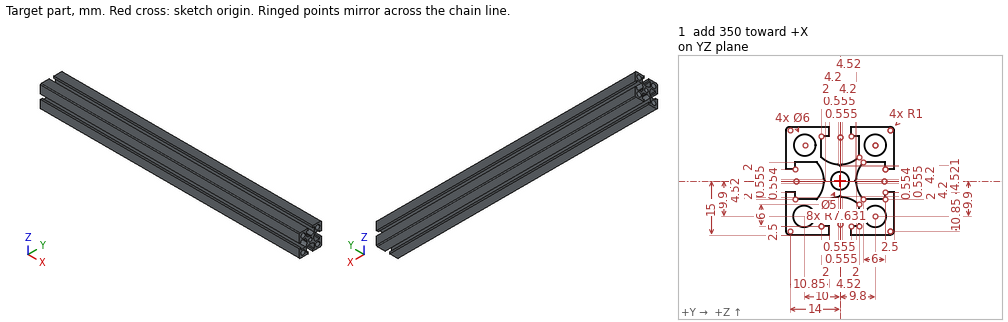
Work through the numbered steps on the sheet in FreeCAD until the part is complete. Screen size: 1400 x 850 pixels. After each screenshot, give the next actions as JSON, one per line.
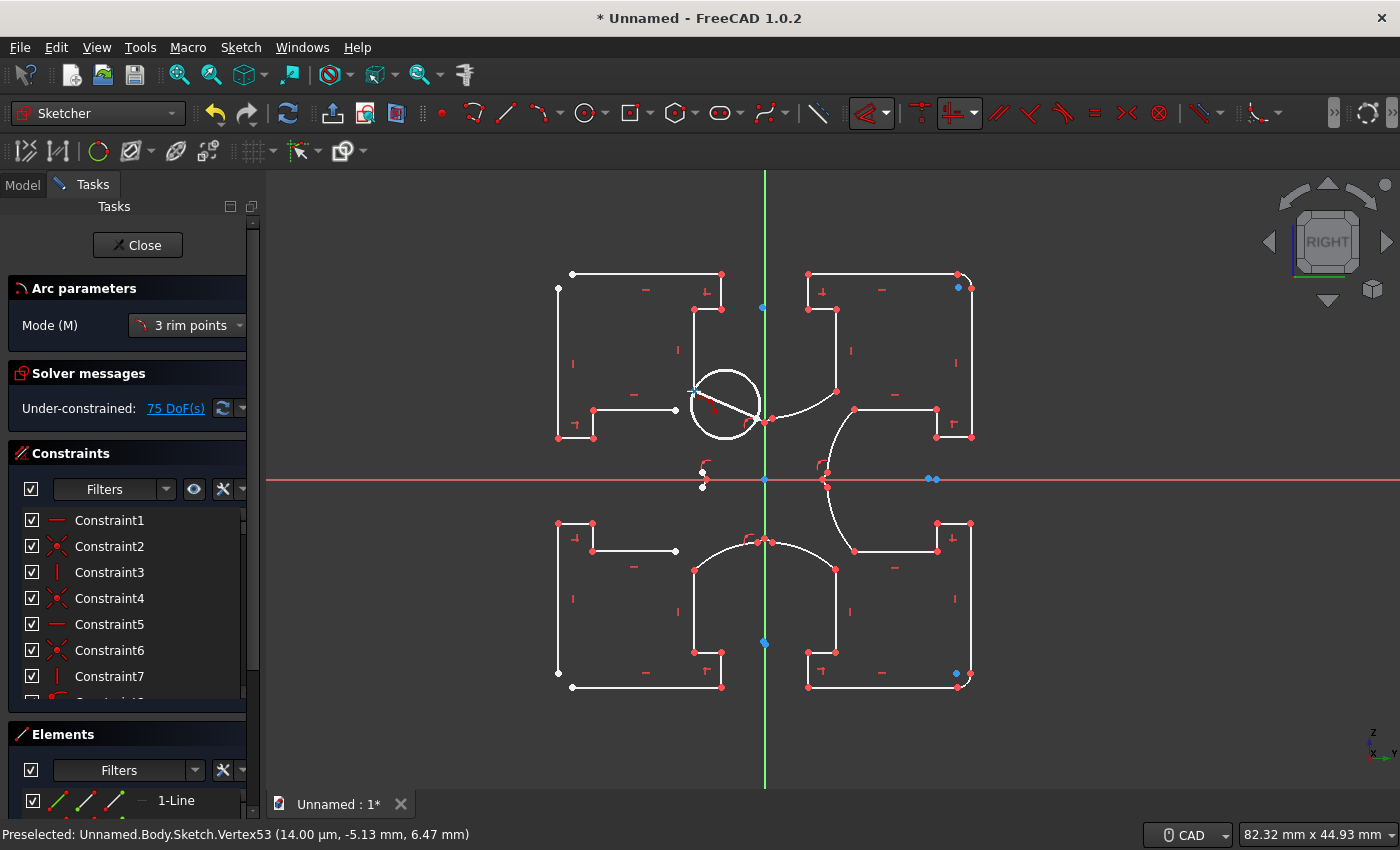
{"action": "scroll", "coordinate": [723, 409], "scroll_direction": "up", "scroll_amount": 6}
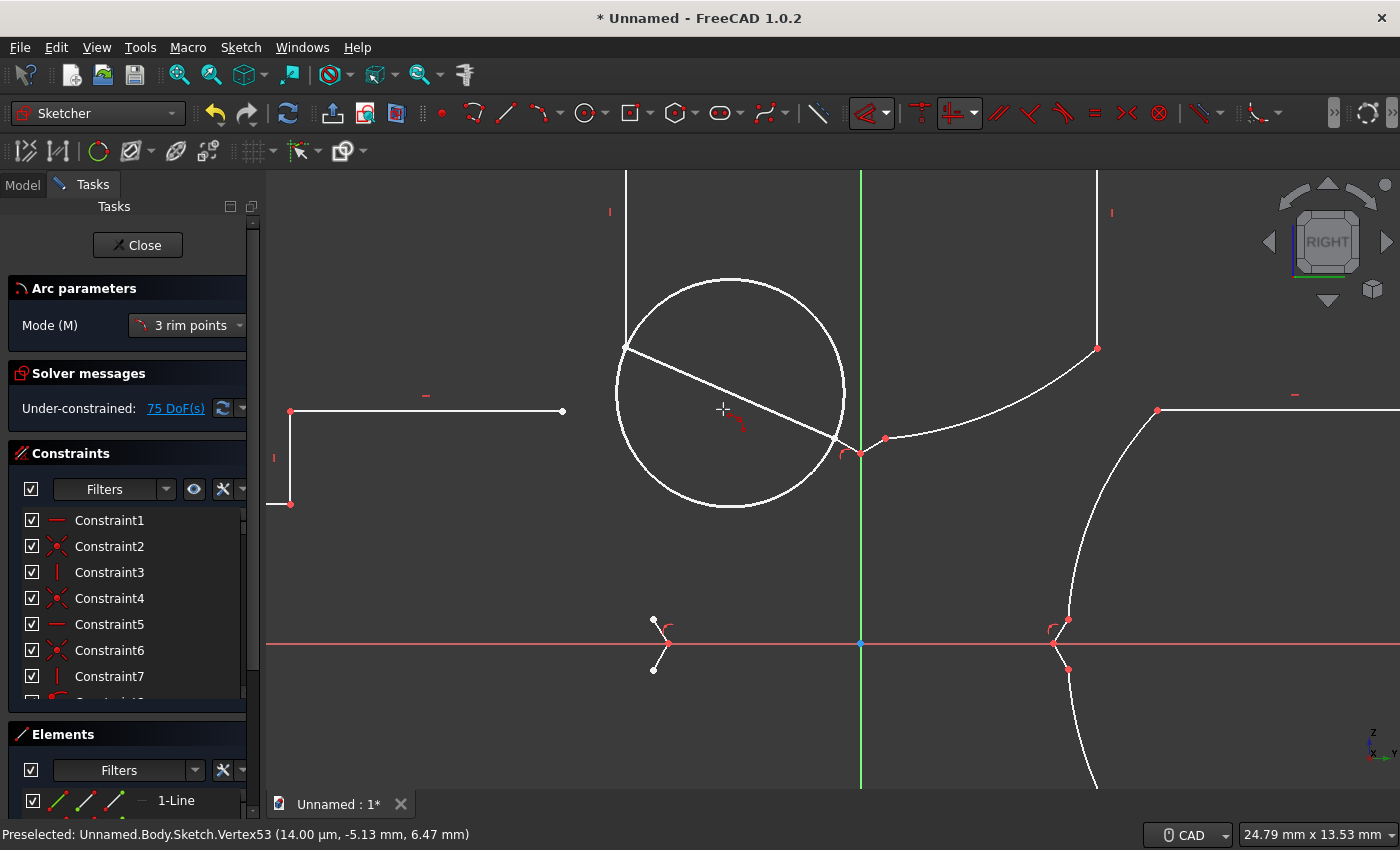
{"action": "left_click", "coordinate": [723, 409]}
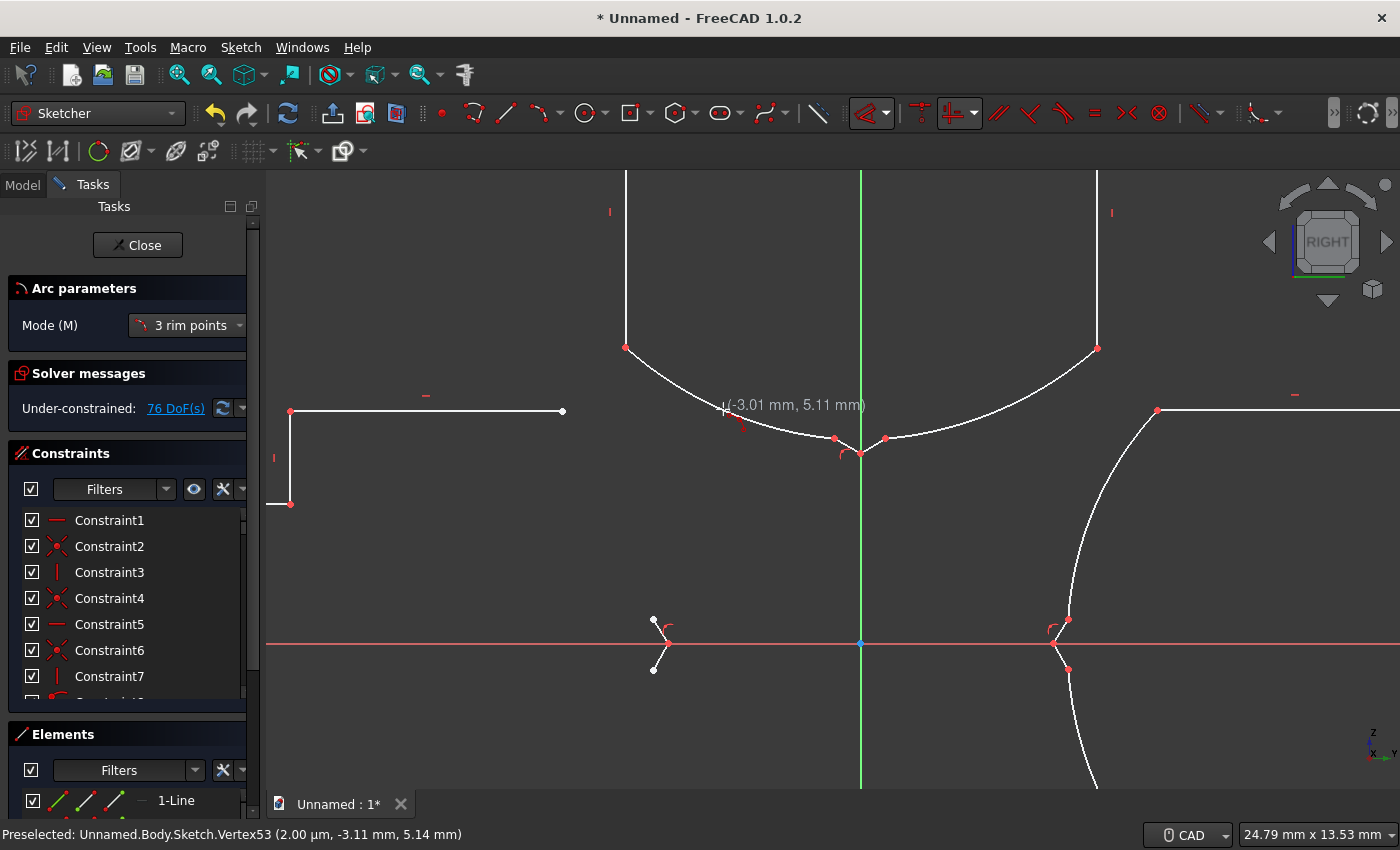
{"action": "scroll", "coordinate": [723, 409], "scroll_direction": "down", "scroll_amount": 6}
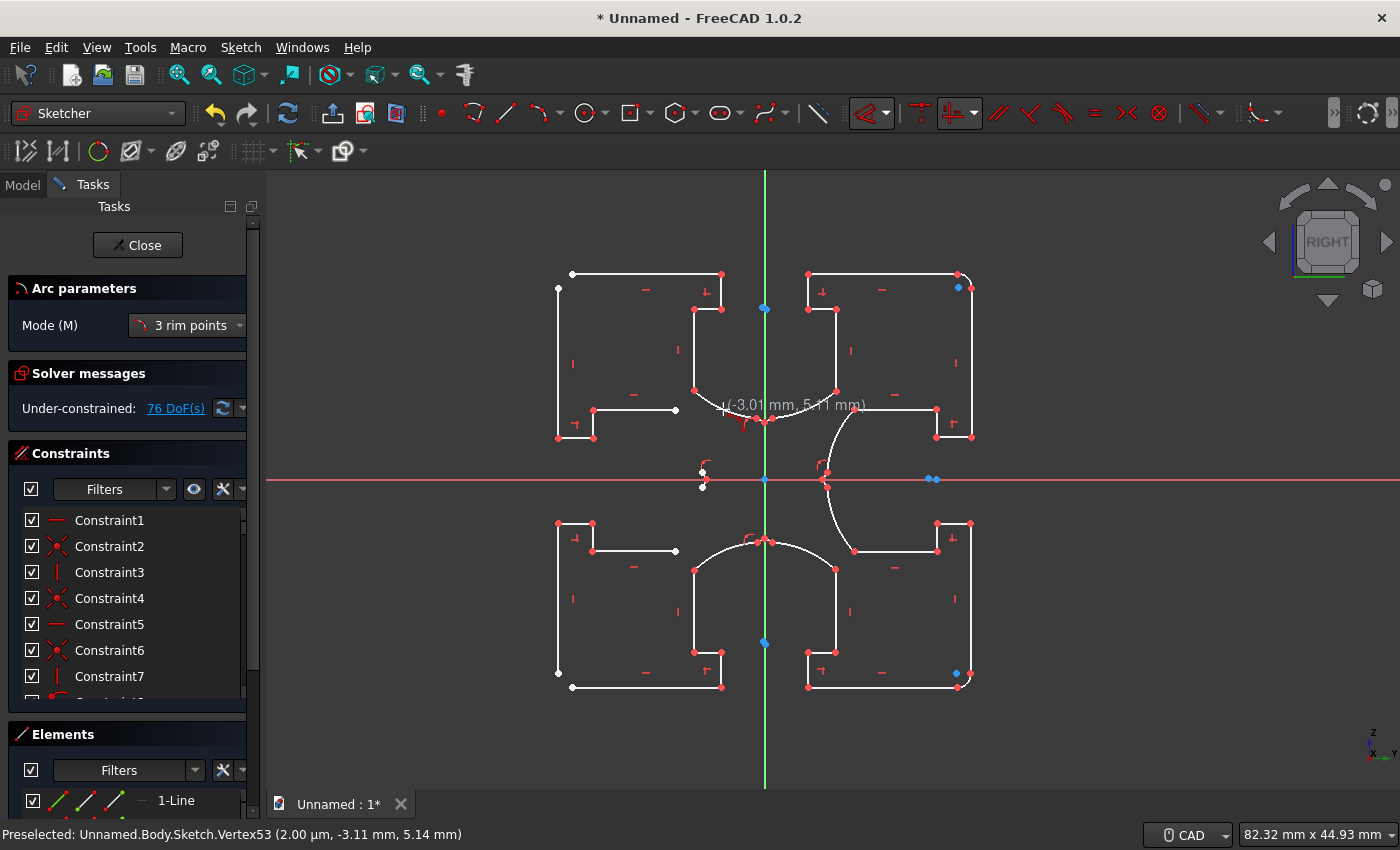
{"action": "left_click", "coordinate": [572, 274]}
{"action": "left_click", "coordinate": [558, 288]}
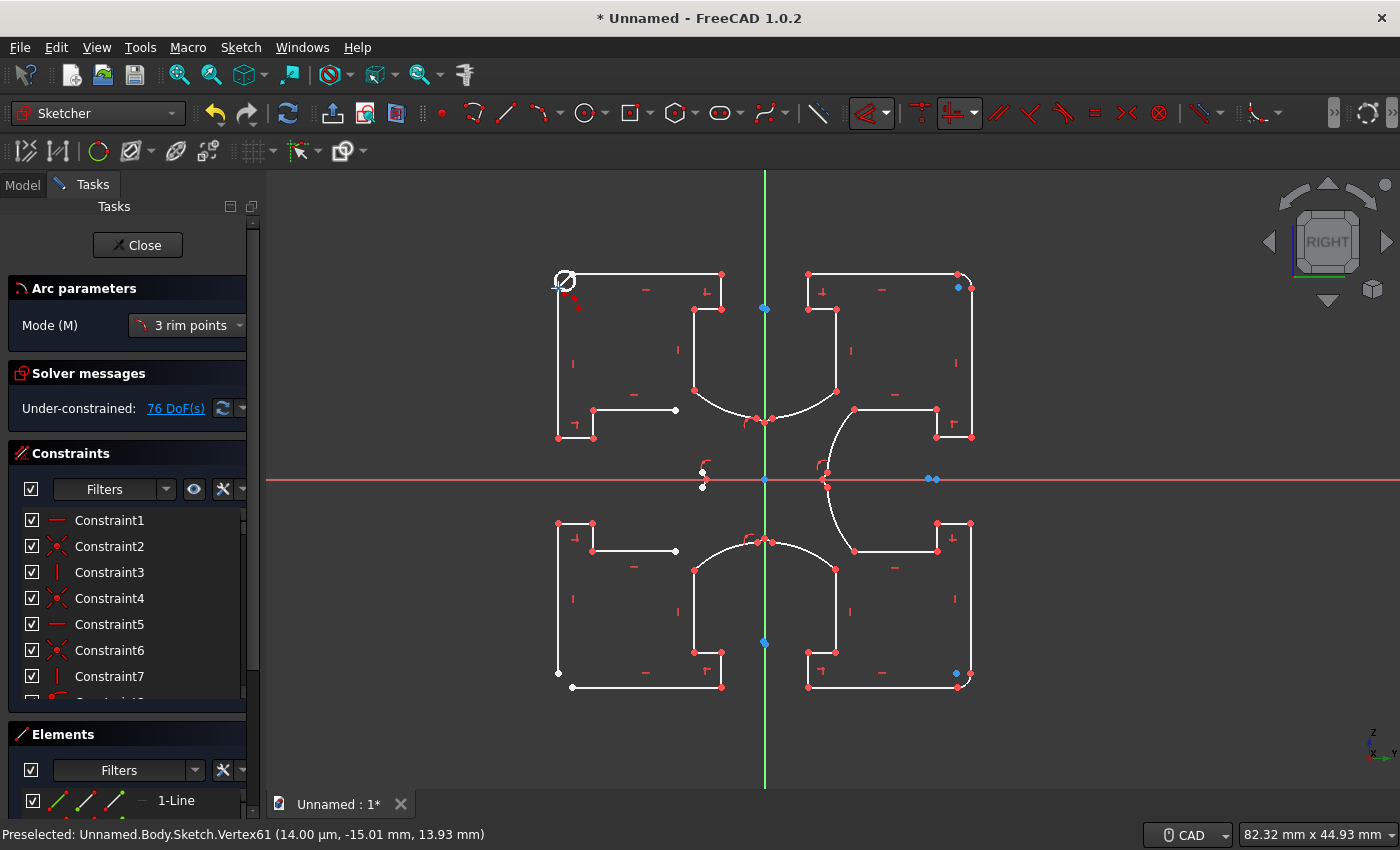
{"action": "scroll", "coordinate": [562, 277], "scroll_direction": "up", "scroll_amount": 7}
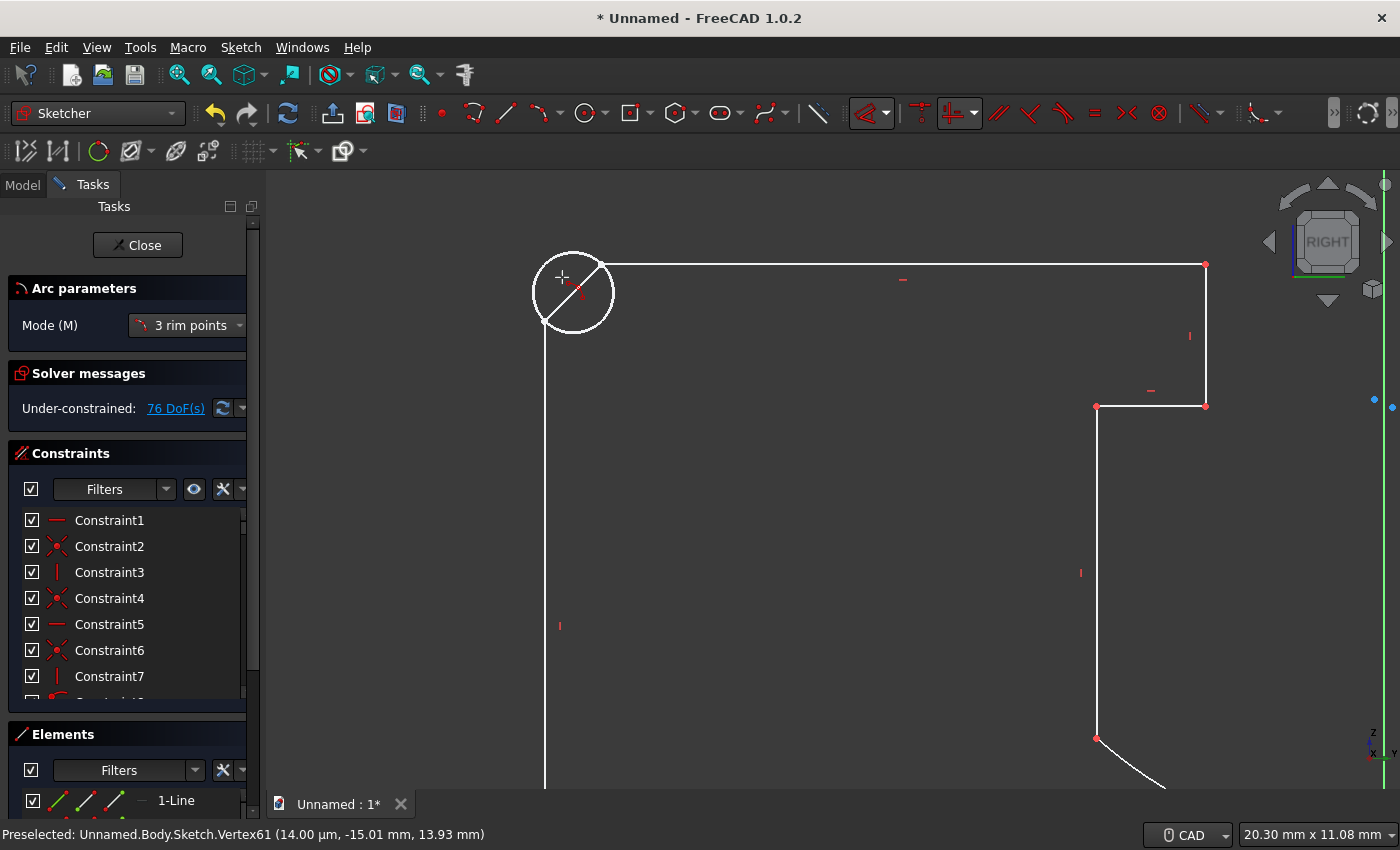
{"action": "left_click", "coordinate": [562, 278]}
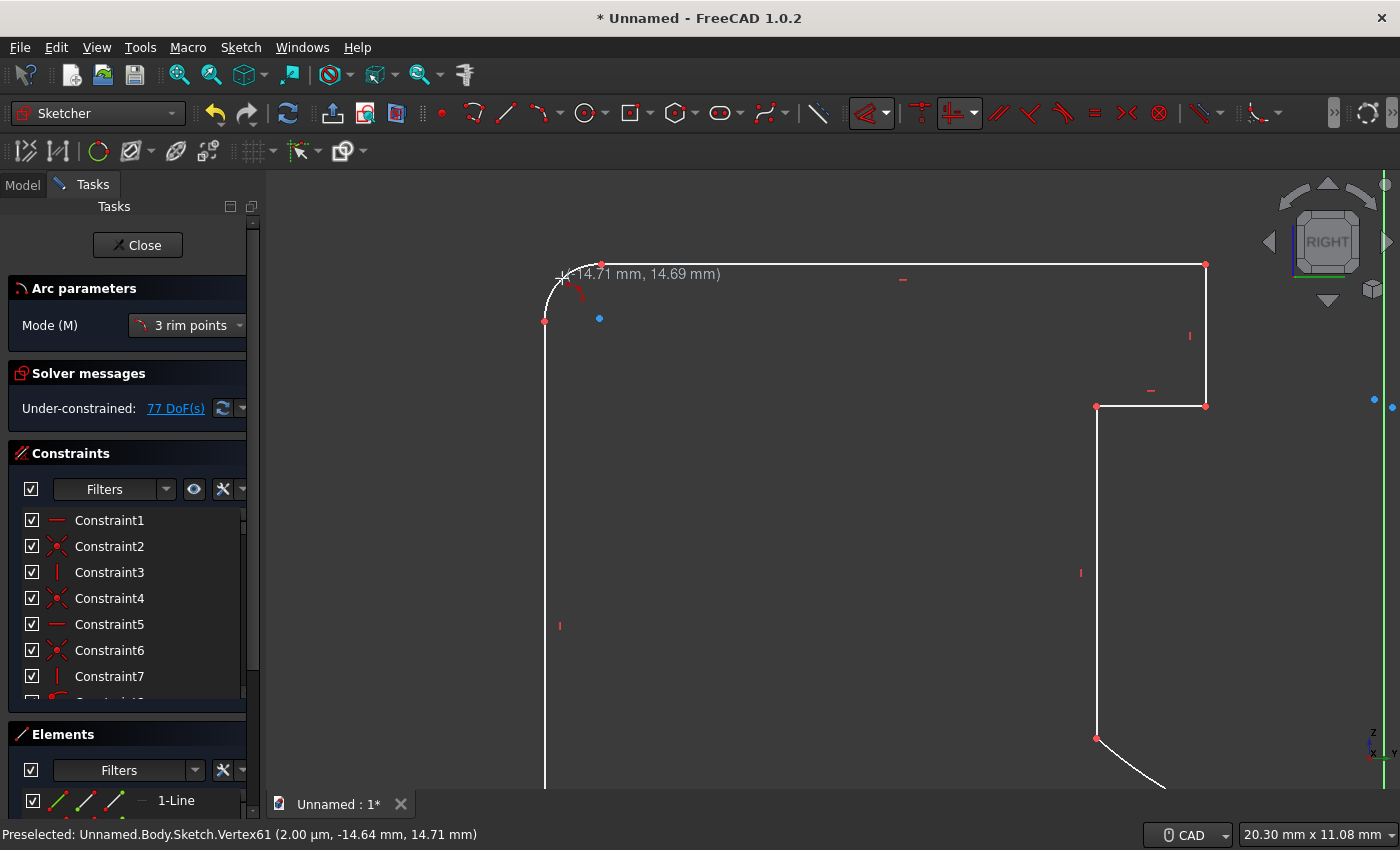
{"action": "scroll", "coordinate": [562, 277], "scroll_direction": "down", "scroll_amount": 7}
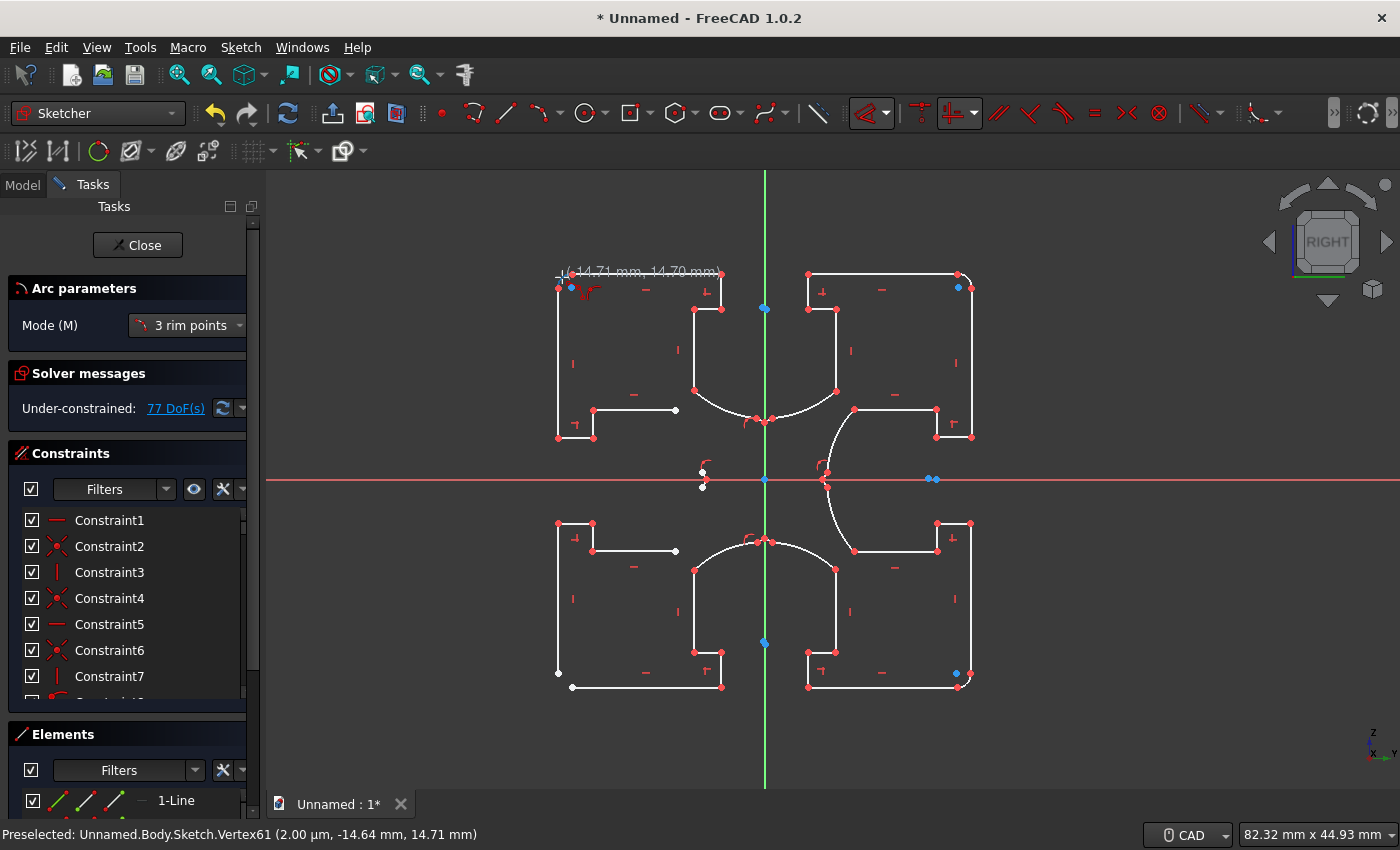
{"action": "left_click", "coordinate": [675, 410]}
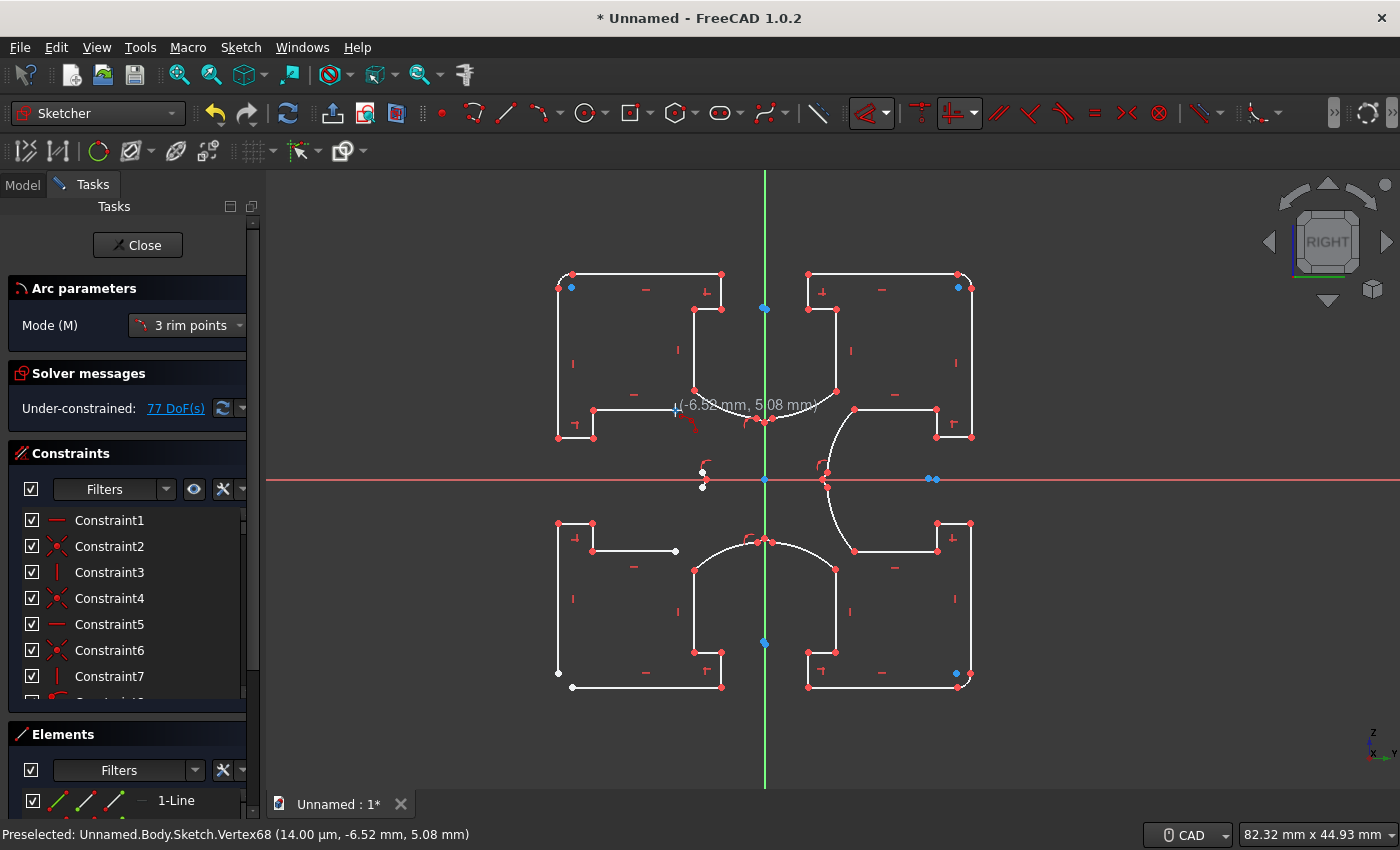
{"action": "scroll", "coordinate": [703, 472], "scroll_direction": "up", "scroll_amount": 7}